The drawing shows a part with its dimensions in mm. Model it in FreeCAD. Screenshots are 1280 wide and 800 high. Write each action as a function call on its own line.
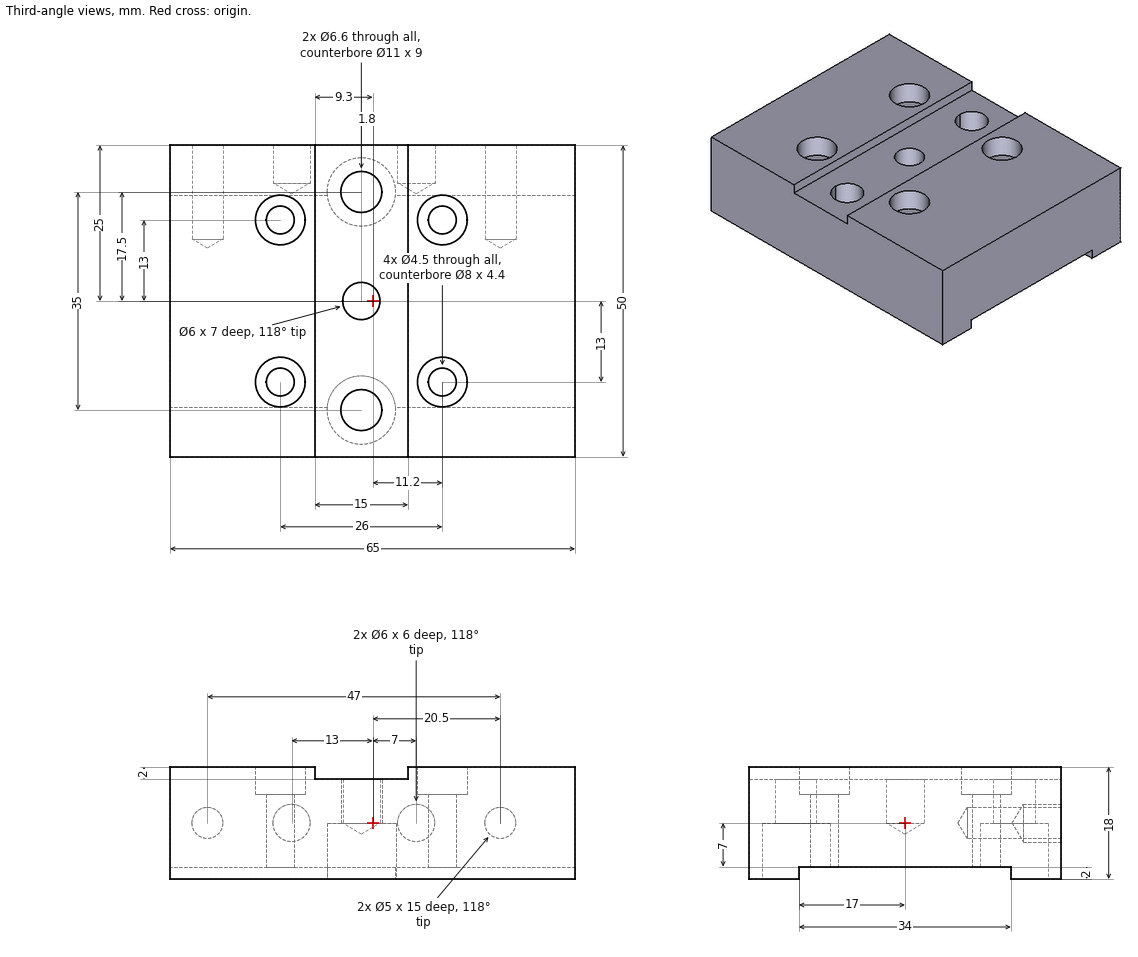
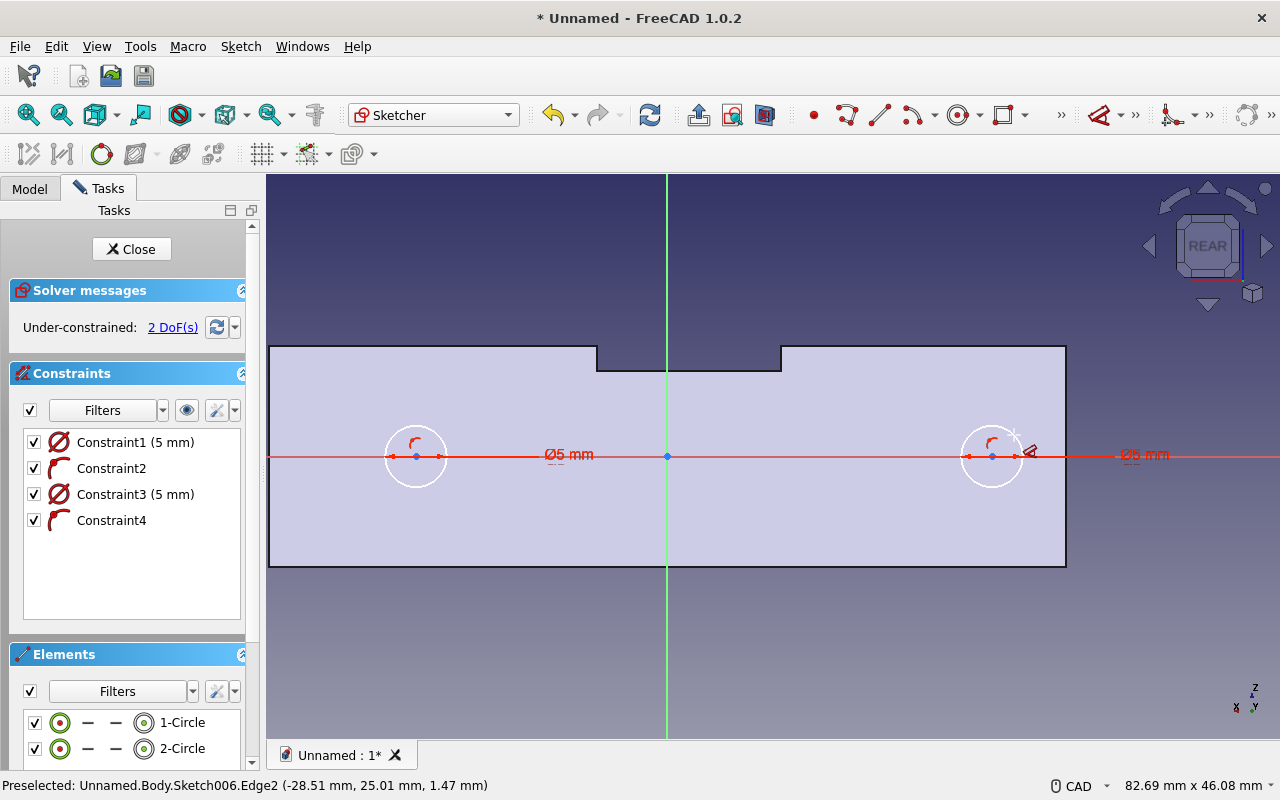
click(416, 456)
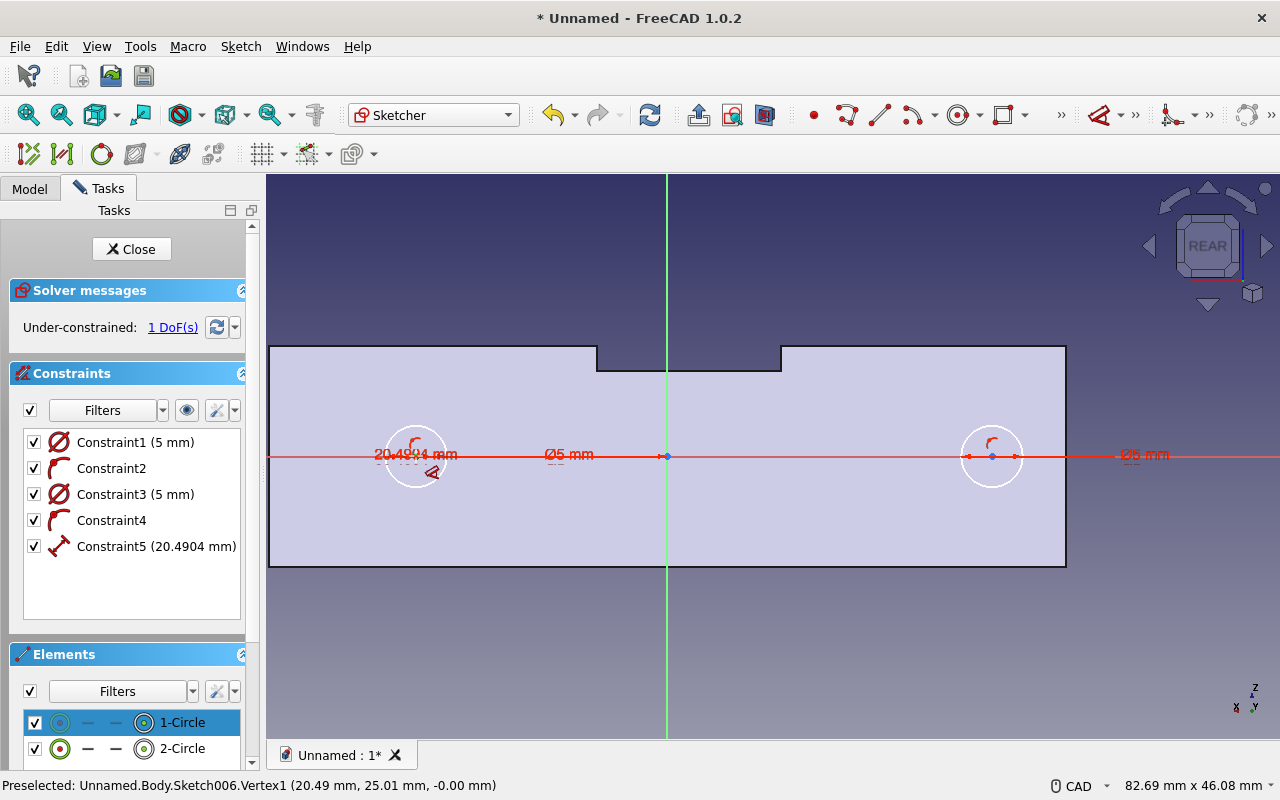
click(992, 456)
click(704, 490)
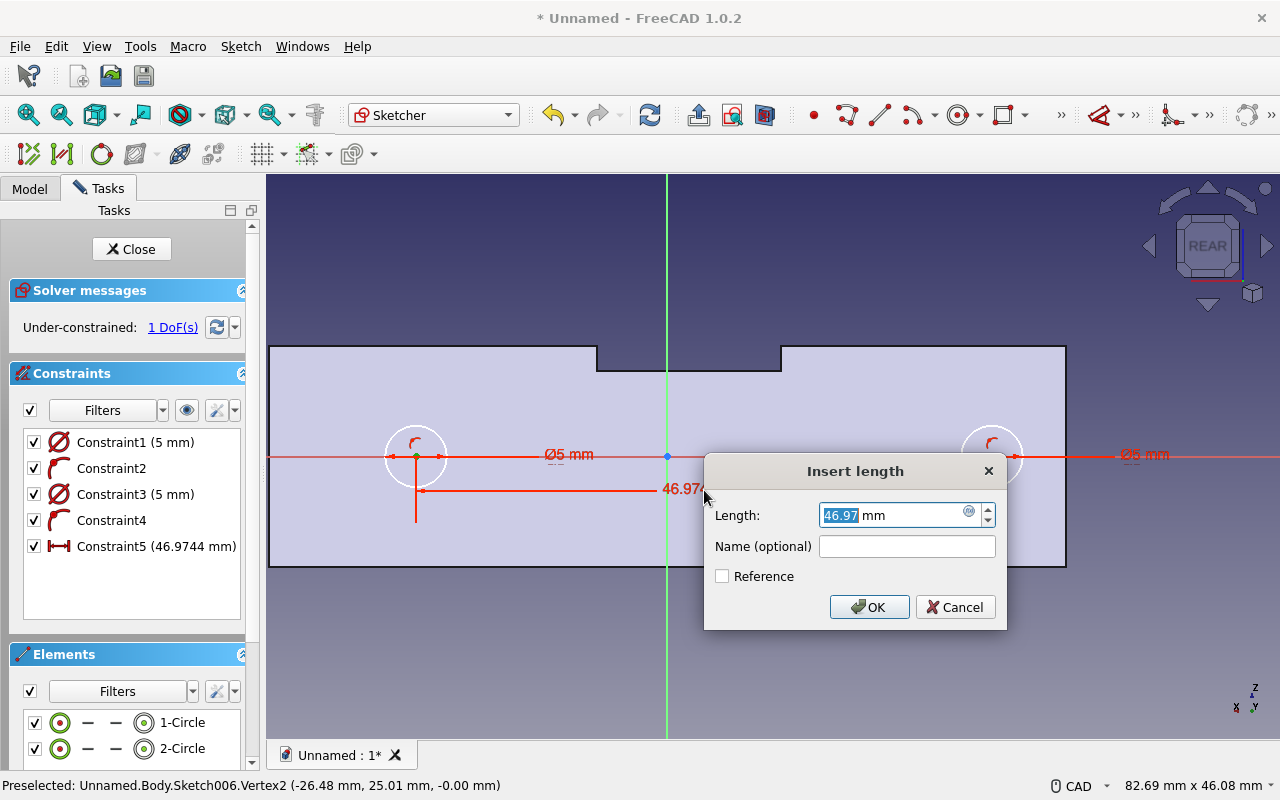
text(47)
key(Return)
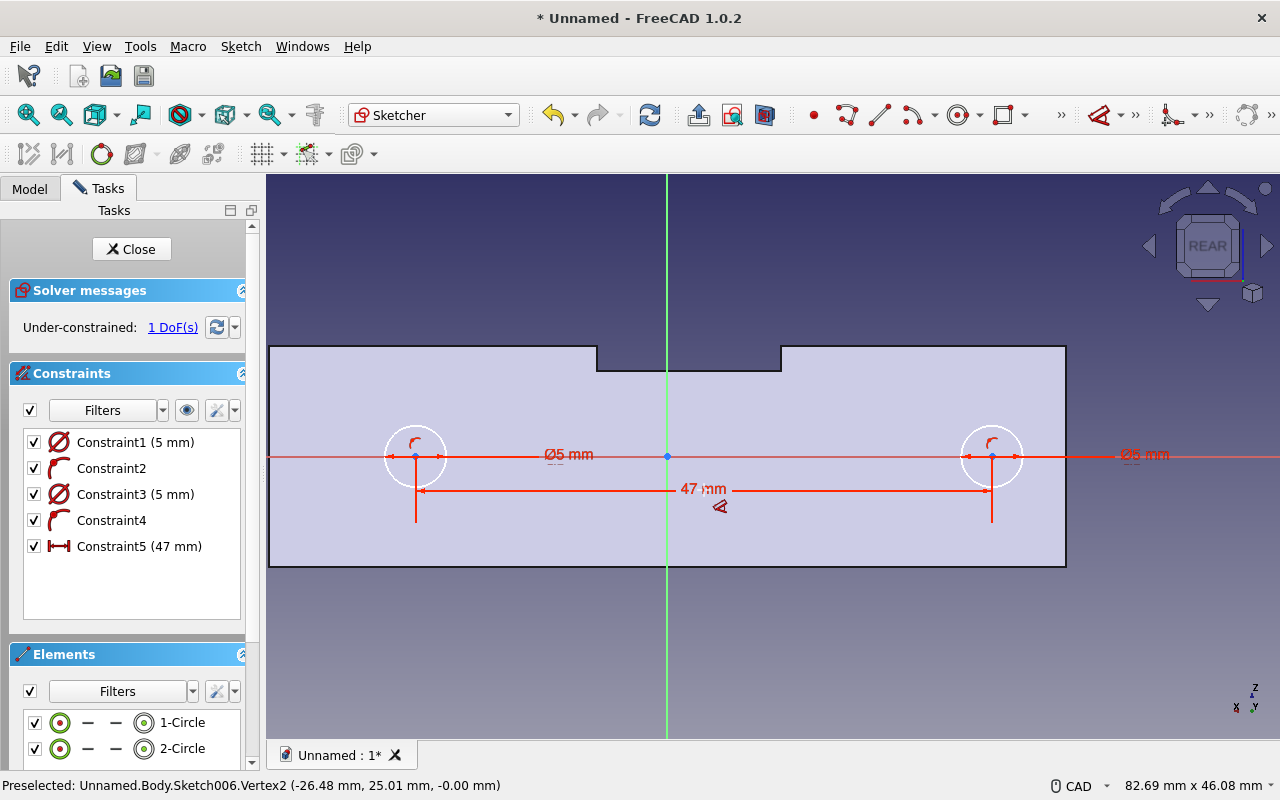
click(416, 456)
click(541, 490)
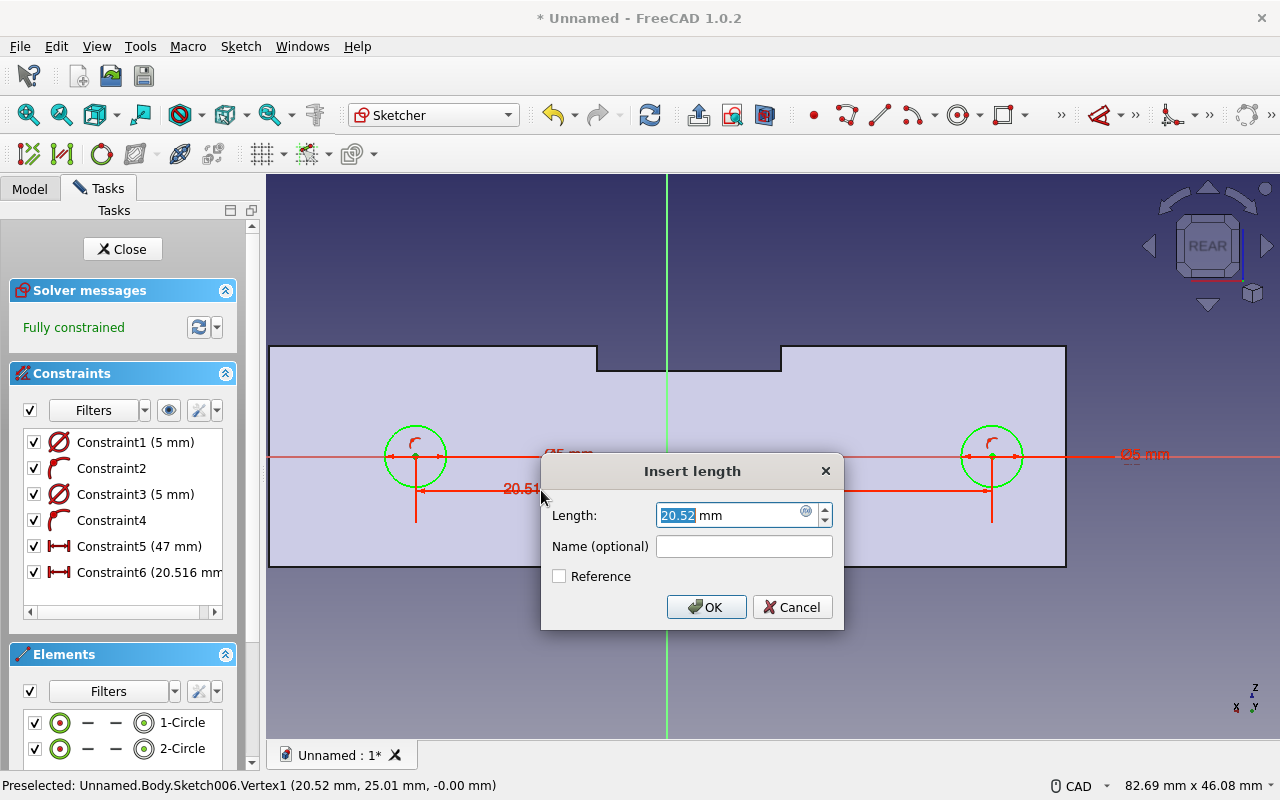
text(20.5)
key(Return)
key(Escape)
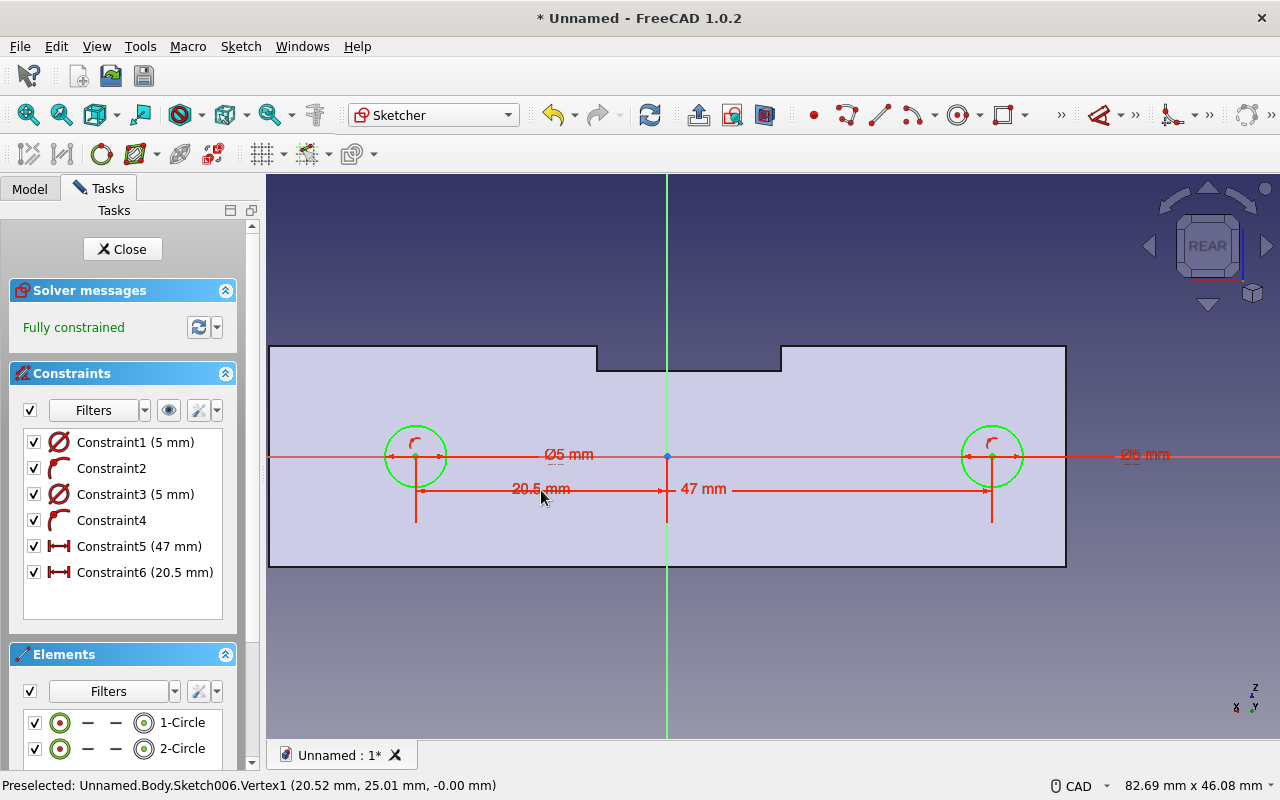
click(123, 249)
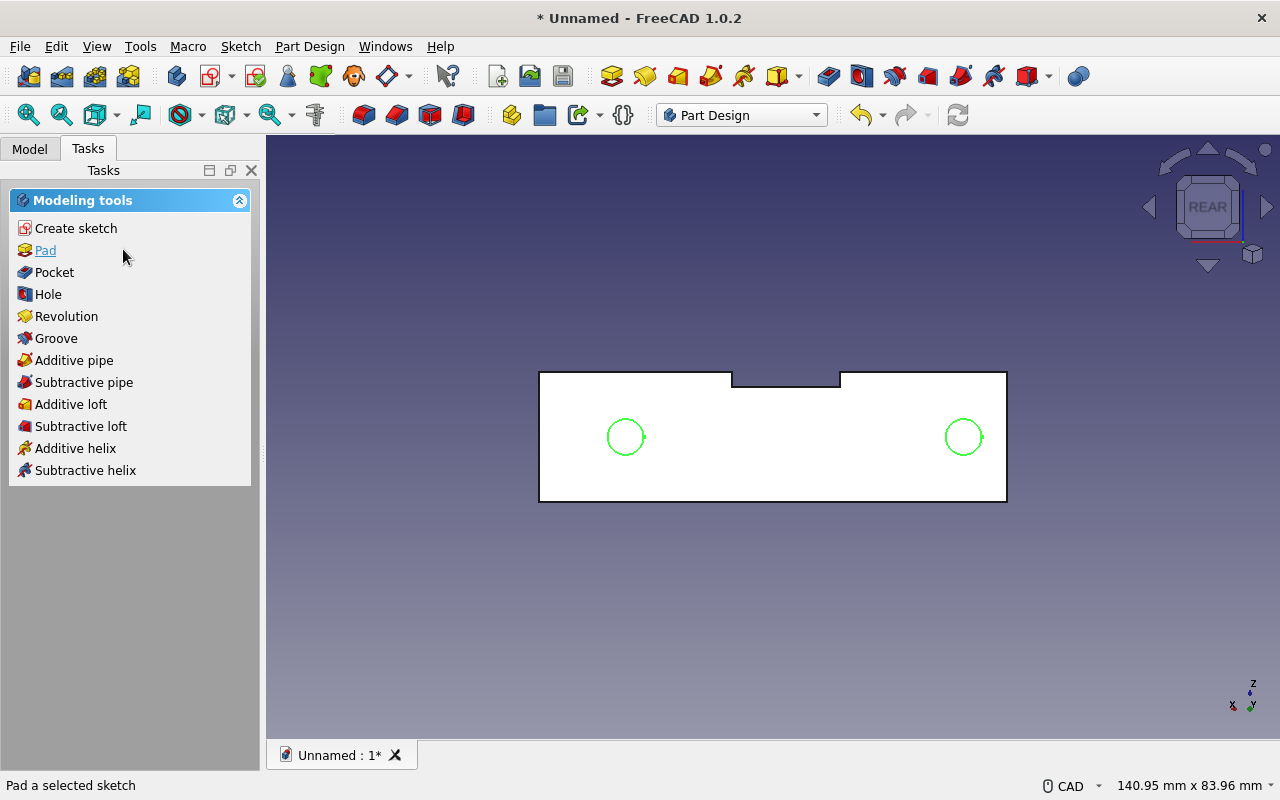
click(862, 76)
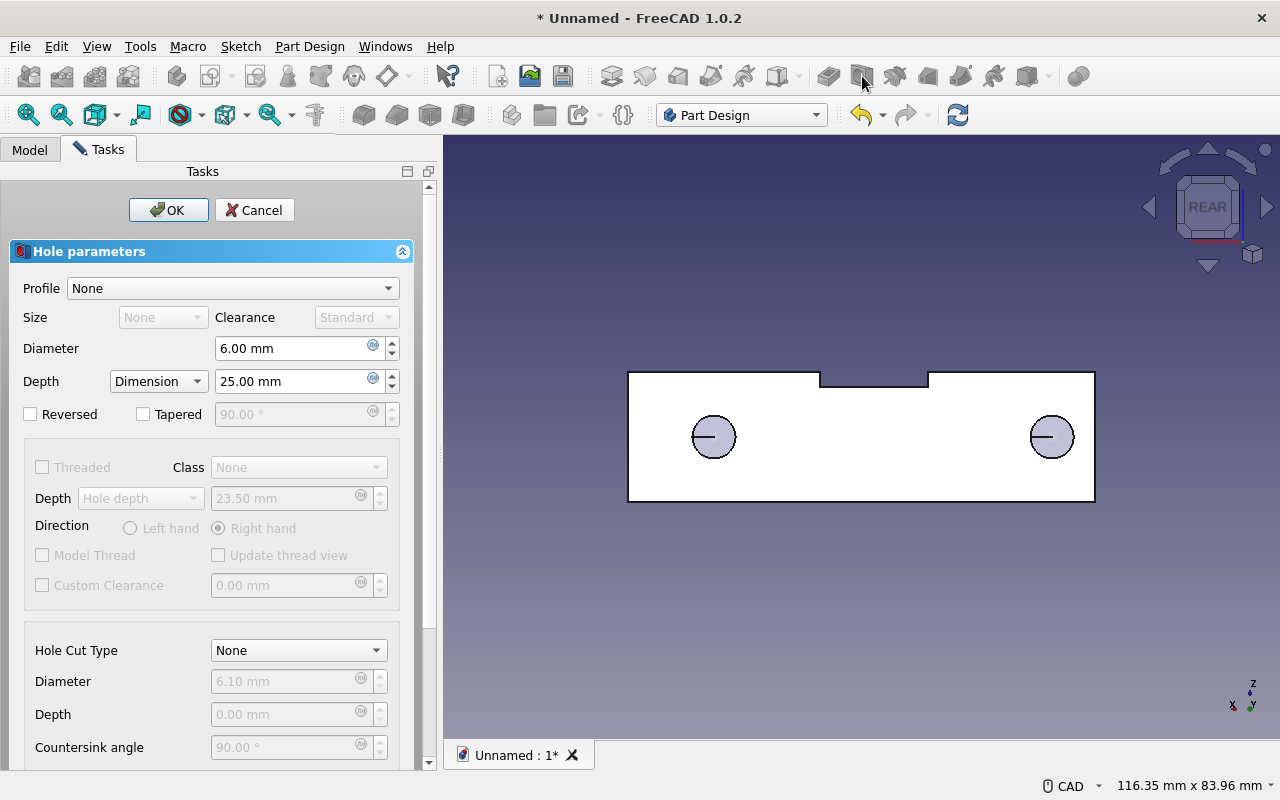
triple_click(300, 348)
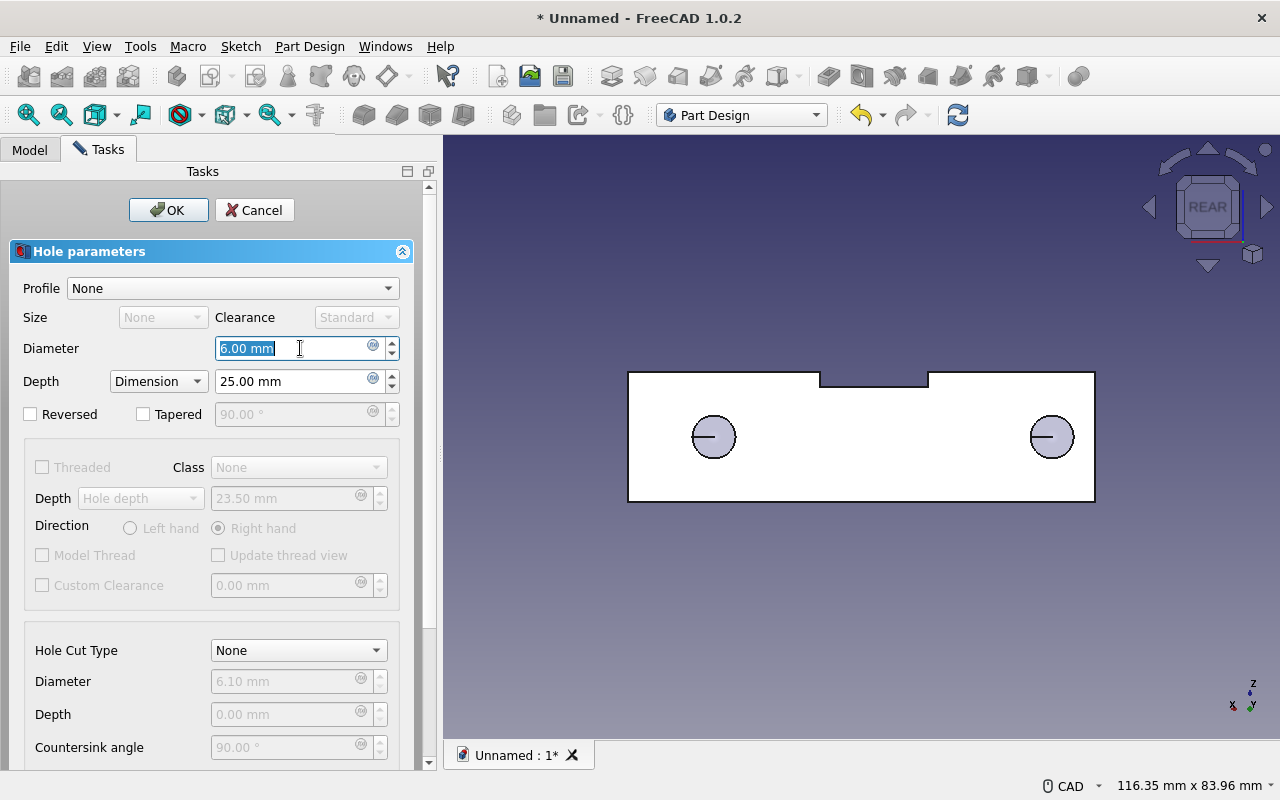
text(5)
key(Tab)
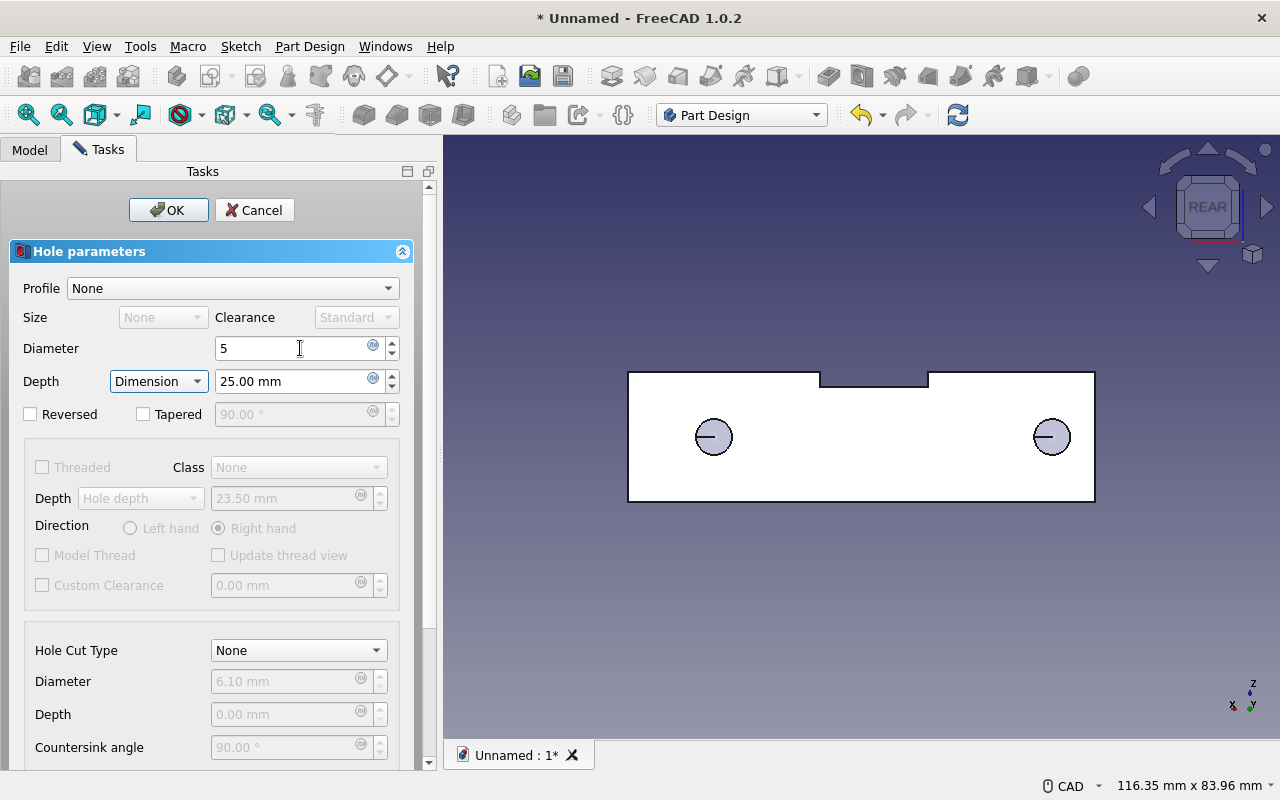
triple_click(300, 382)